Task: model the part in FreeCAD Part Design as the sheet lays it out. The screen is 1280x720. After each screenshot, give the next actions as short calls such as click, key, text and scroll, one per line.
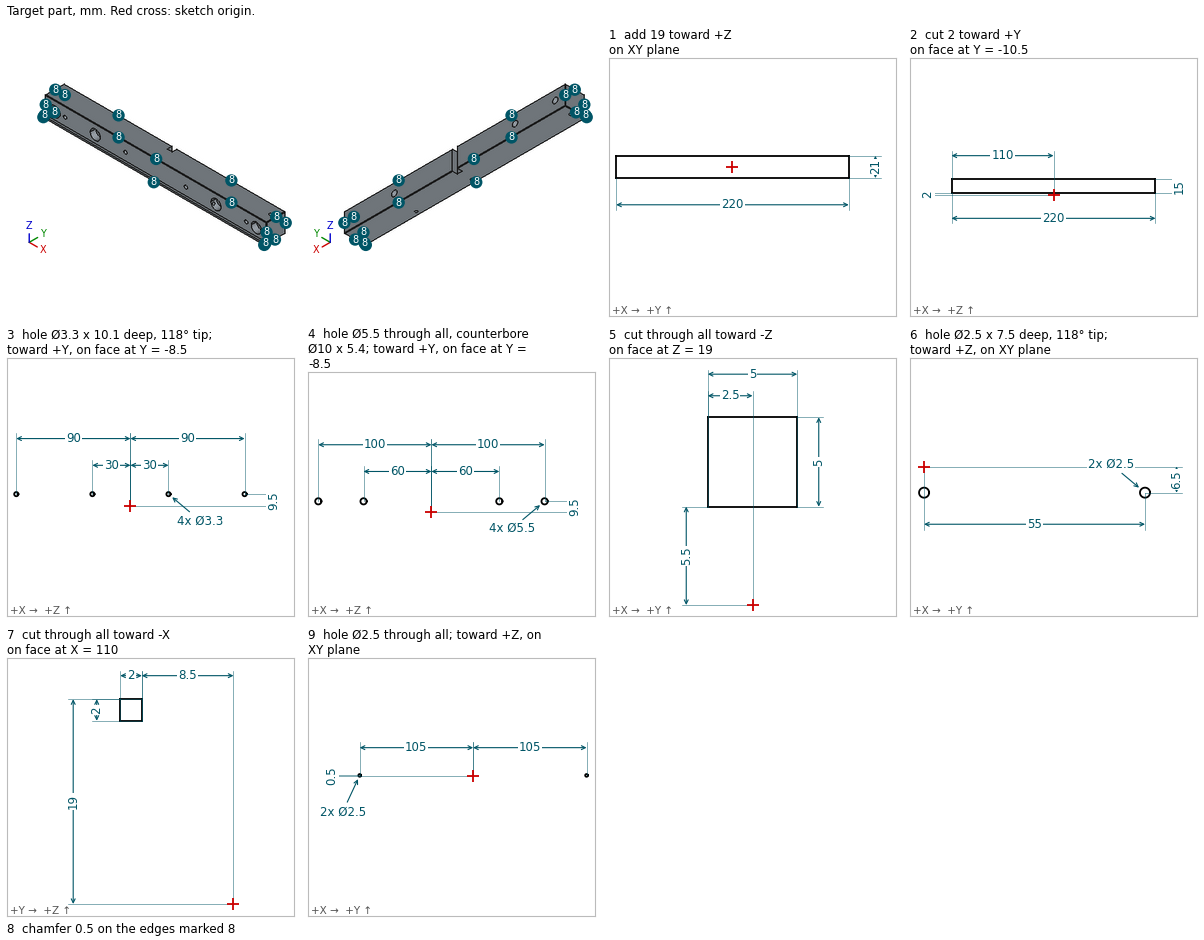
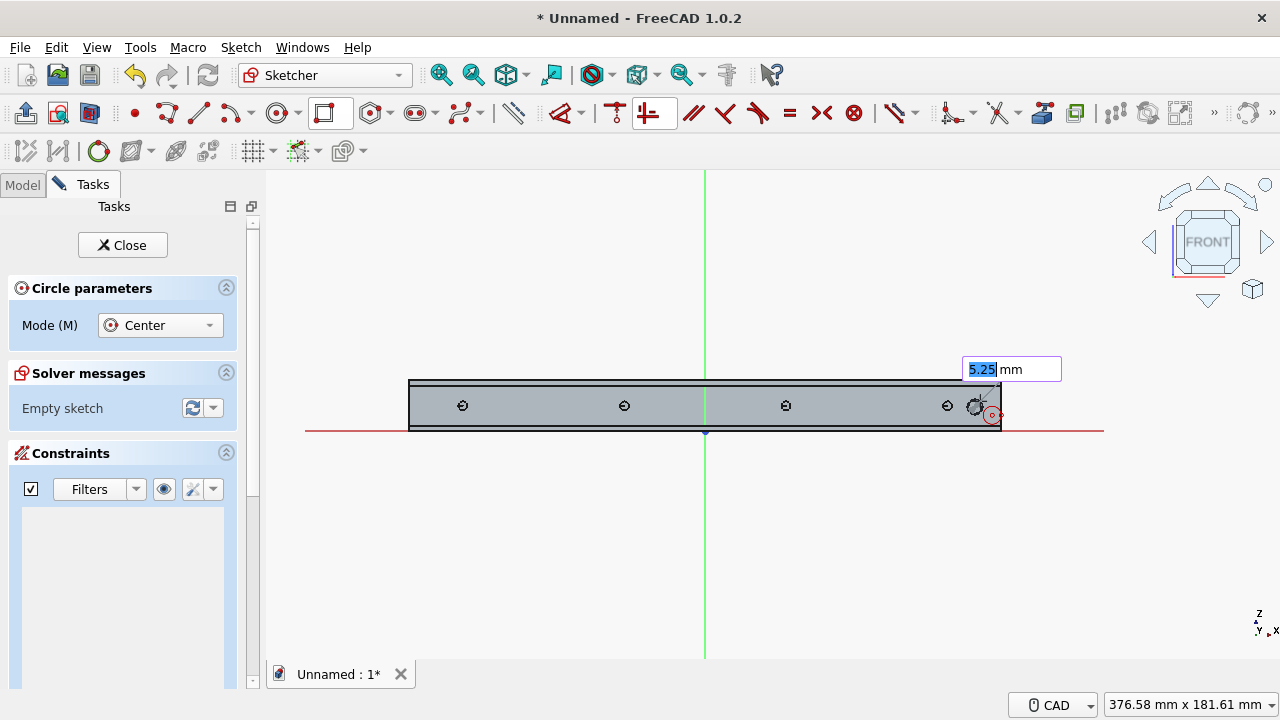
text(5.5)
key(Return)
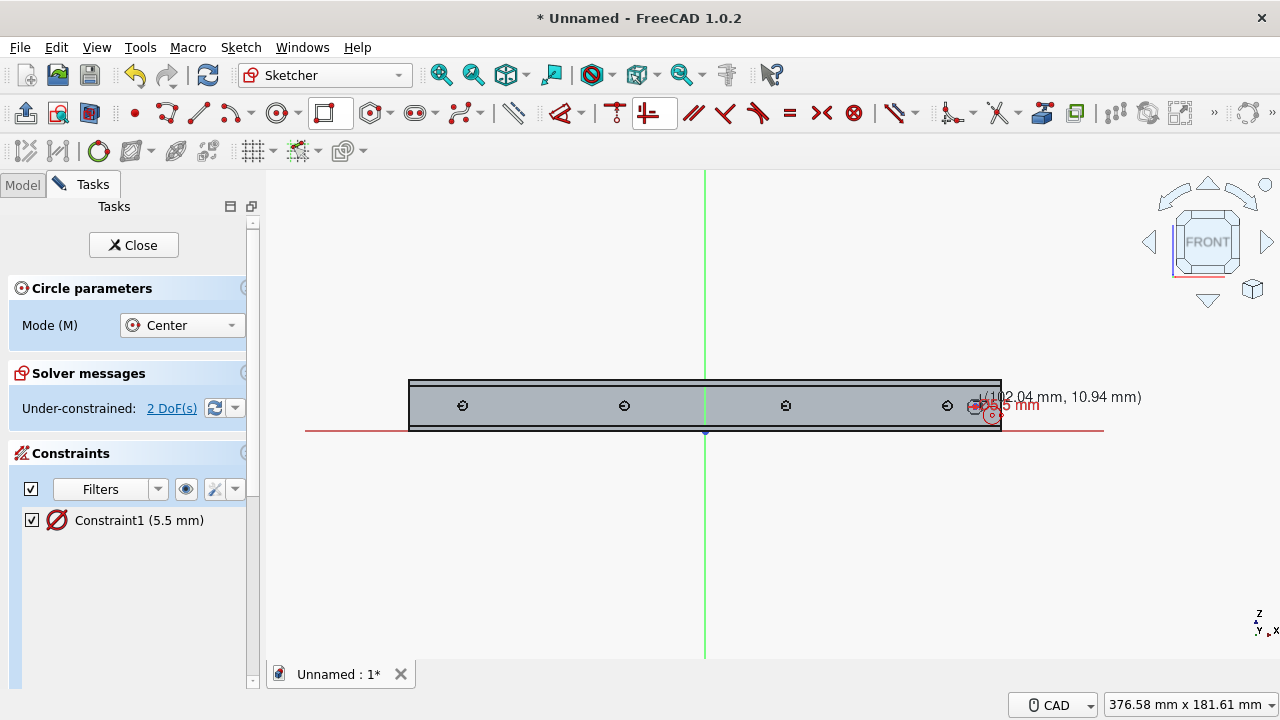
scroll(436, 406, up, 6)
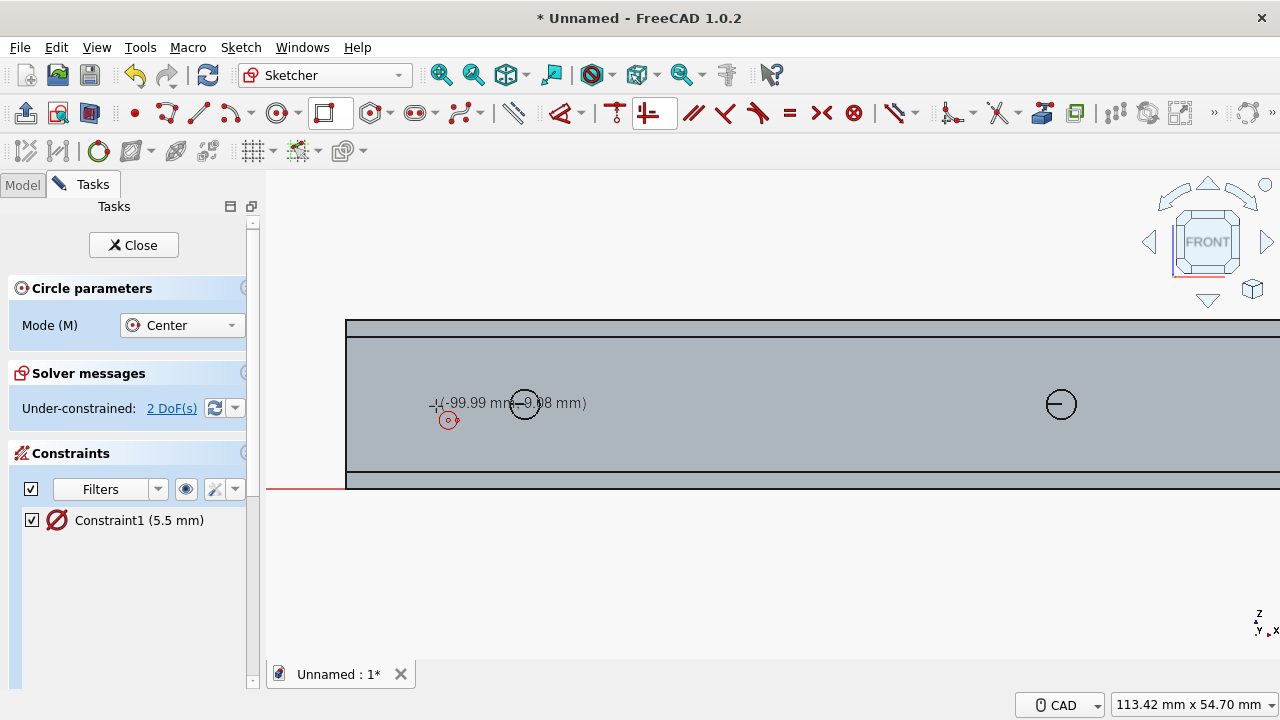
scroll(435, 406, down, 6)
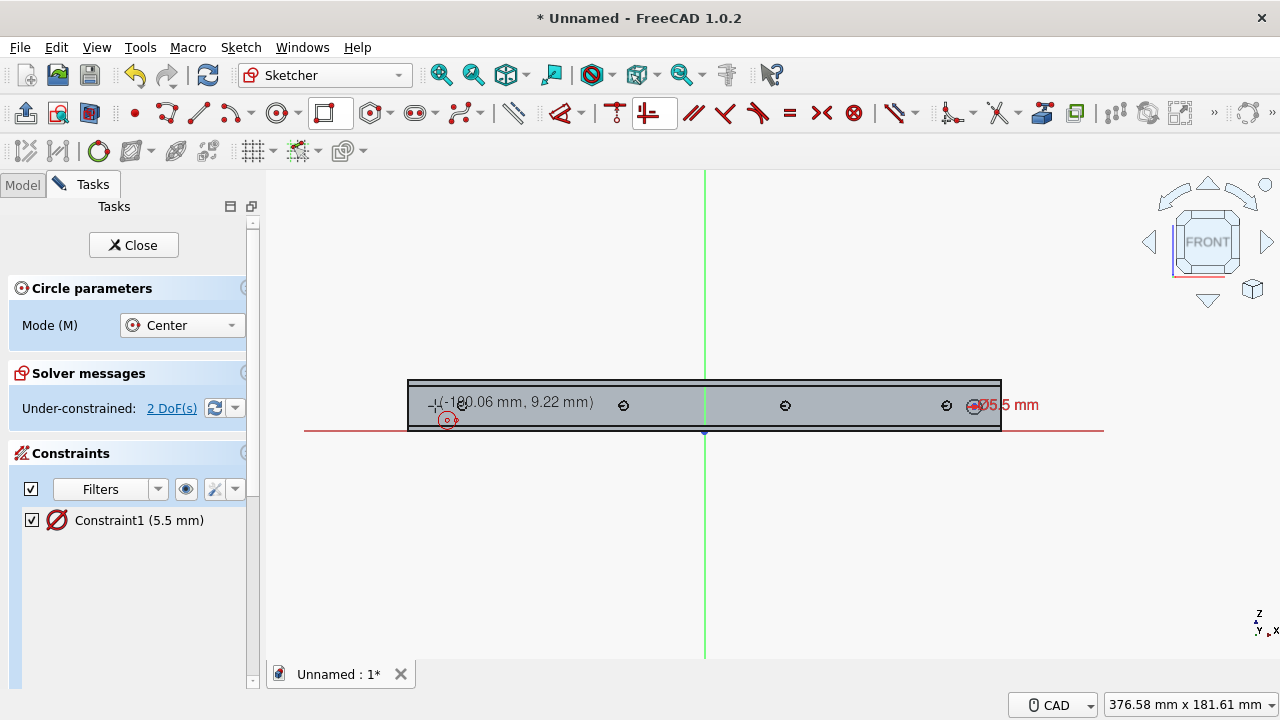
click(435, 406)
move(441, 401)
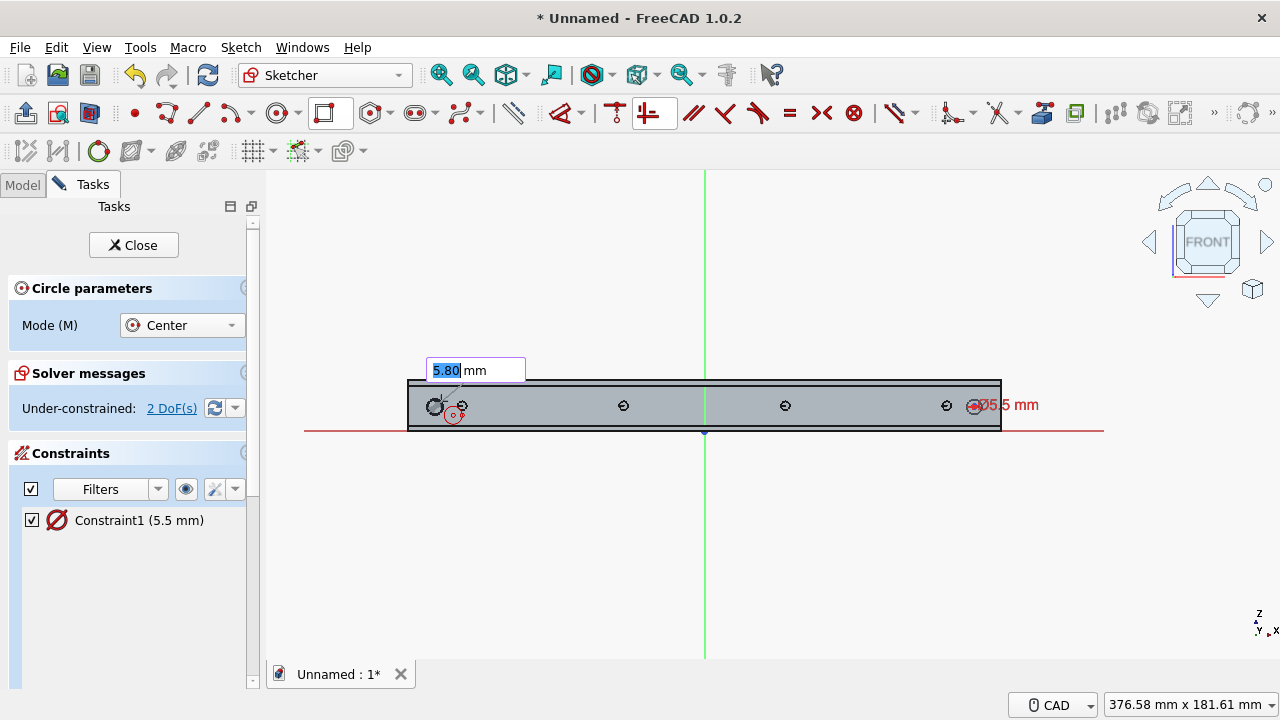
text(5.5)
key(Return)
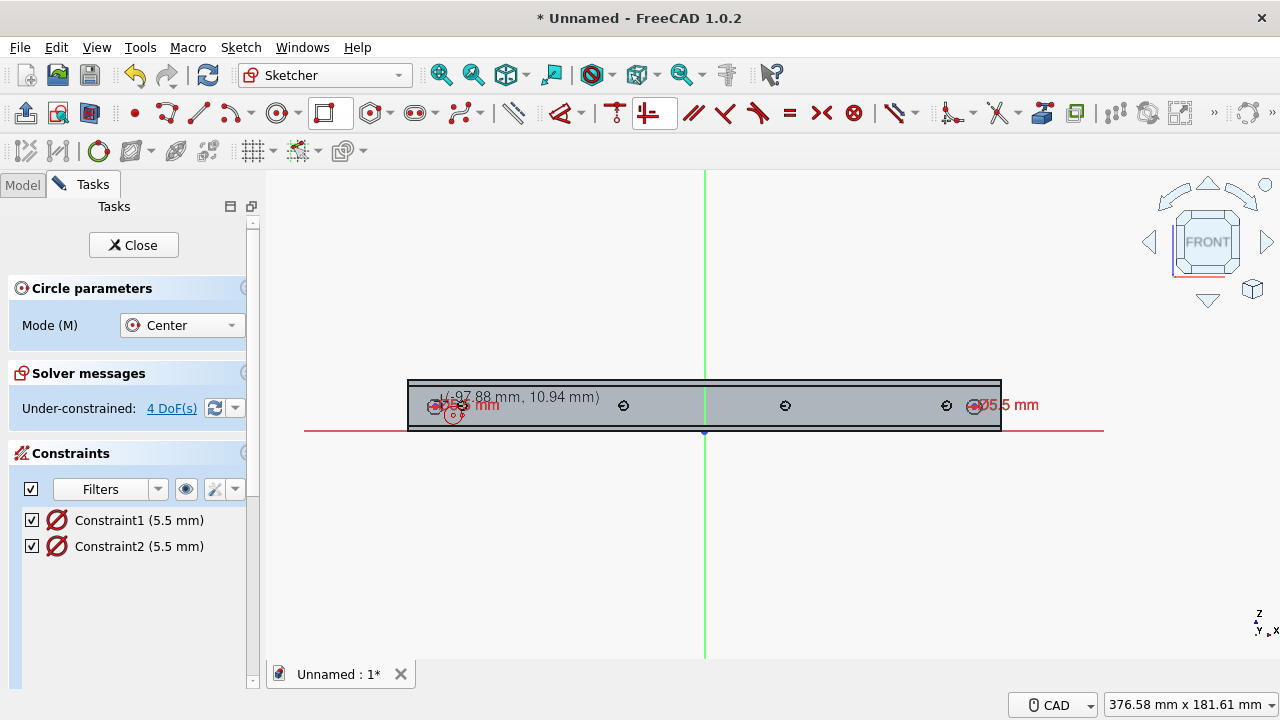
scroll(543, 406, up, 6)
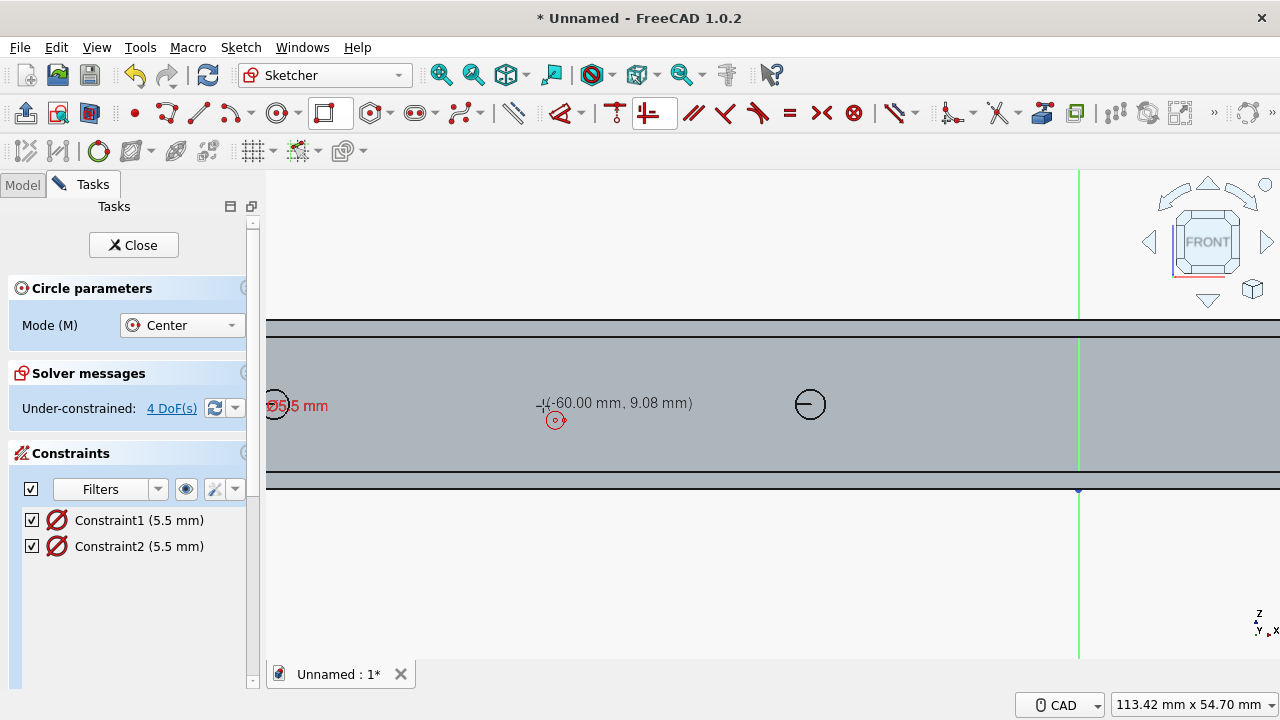
scroll(543, 406, down, 6)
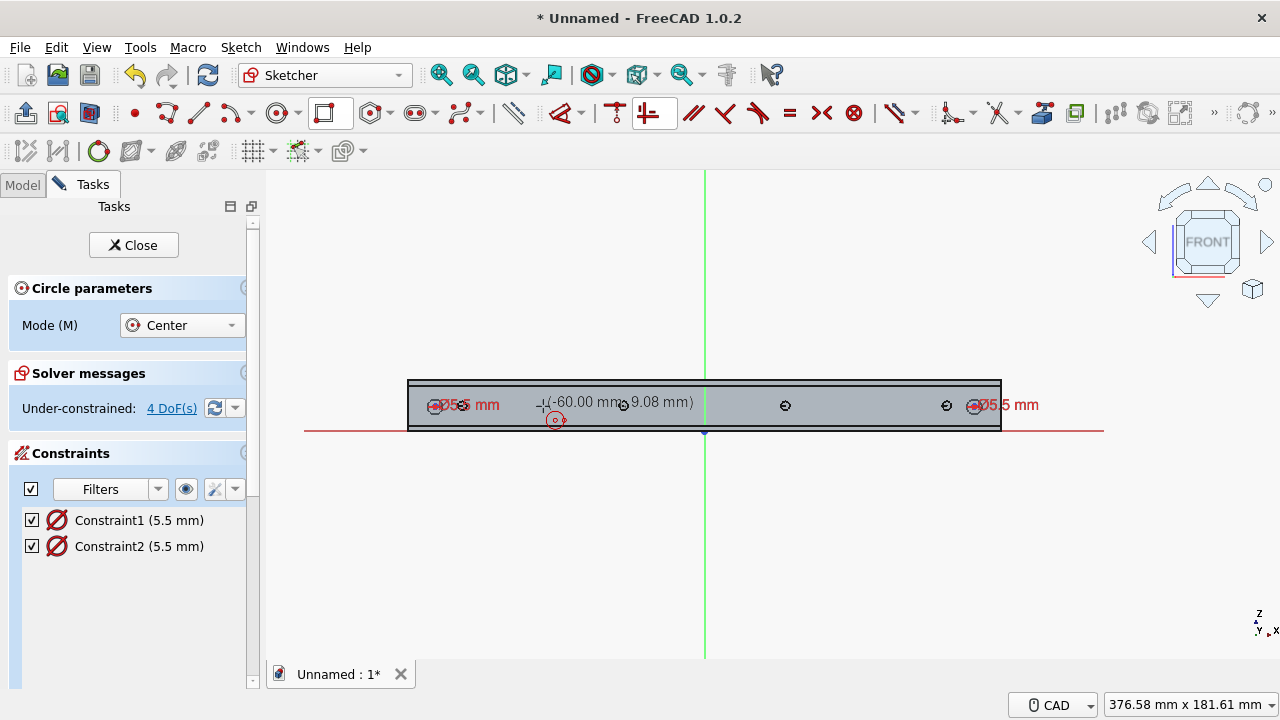
click(543, 406)
move(548, 401)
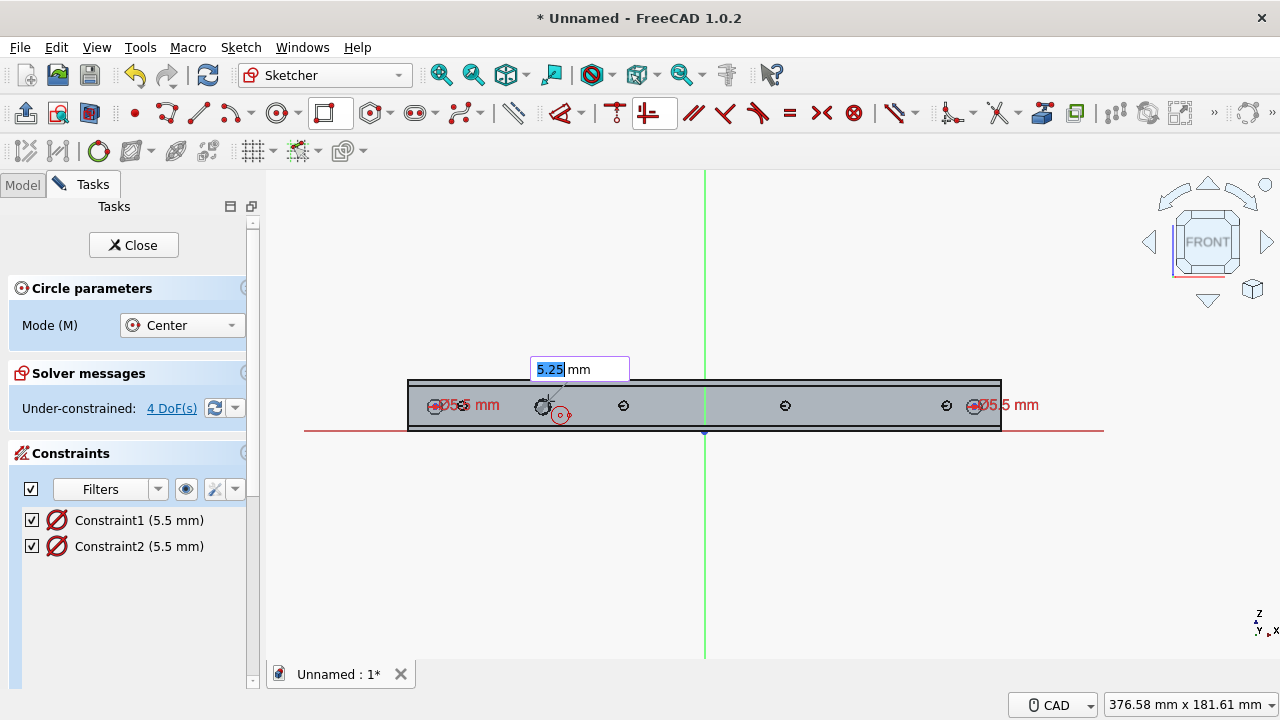
text(5.5)
key(Return)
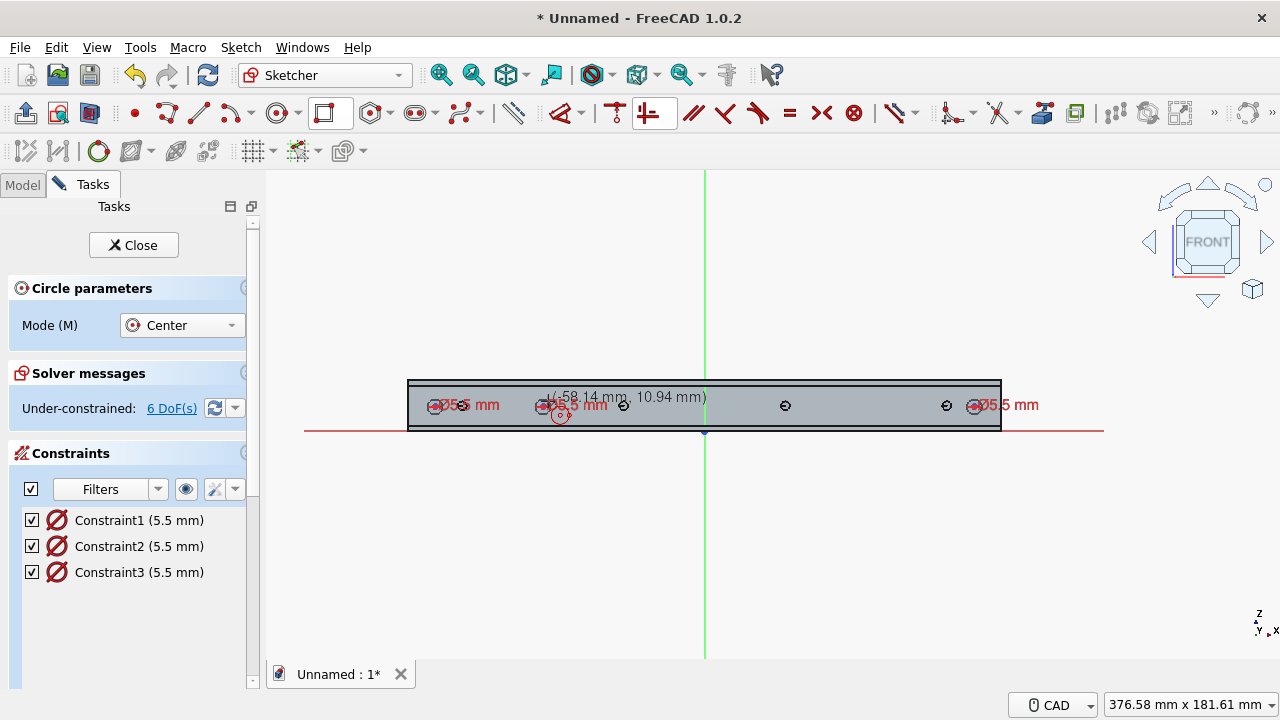
scroll(866, 406, up, 6)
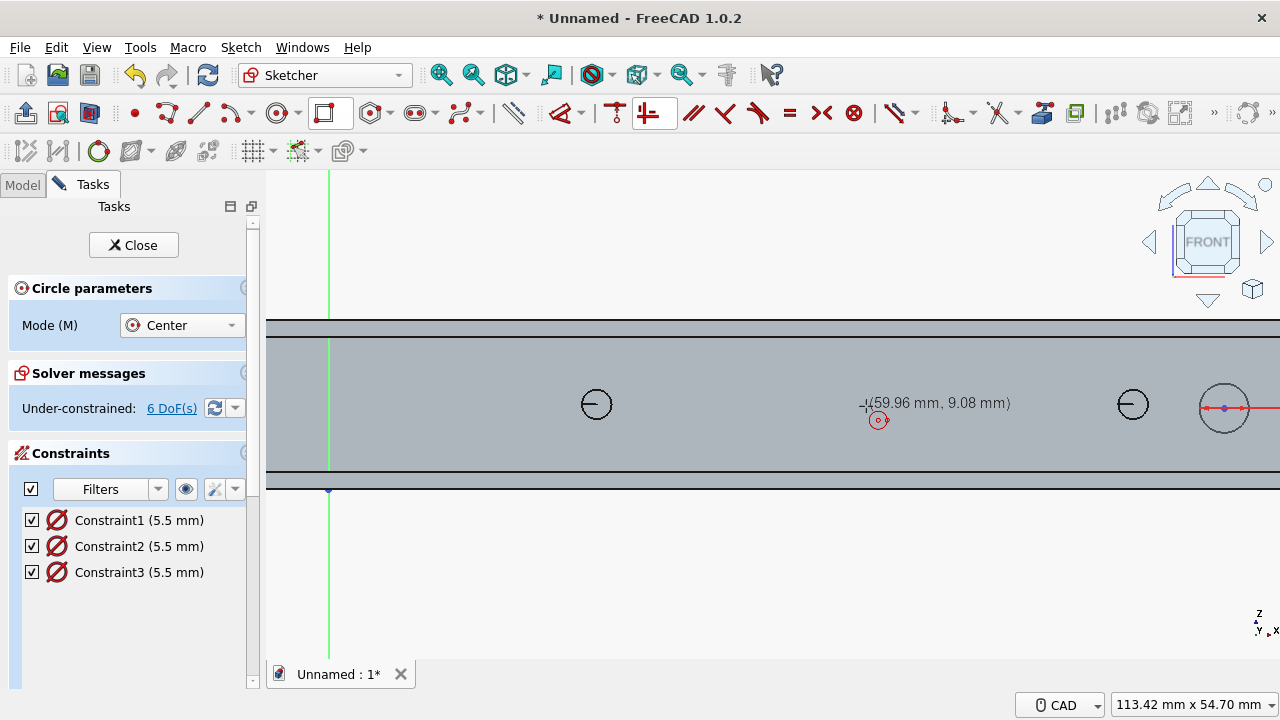
scroll(867, 406, down, 6)